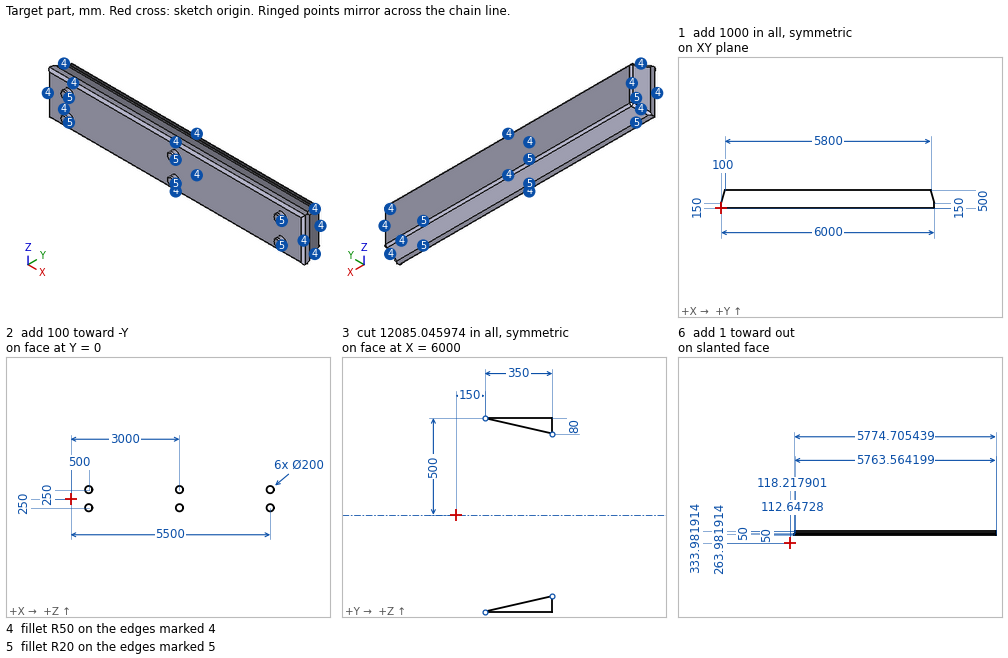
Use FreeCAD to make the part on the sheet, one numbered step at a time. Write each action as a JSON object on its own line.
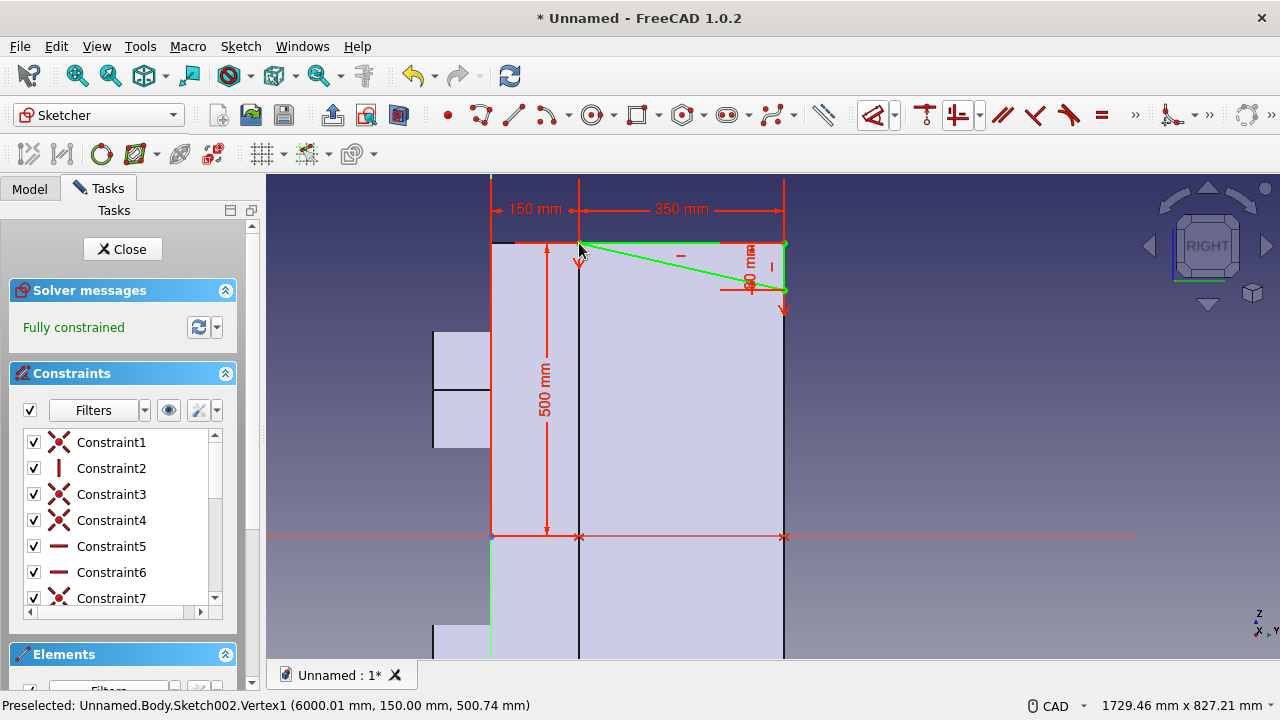
{"action": "left_click", "coordinate": [123, 249]}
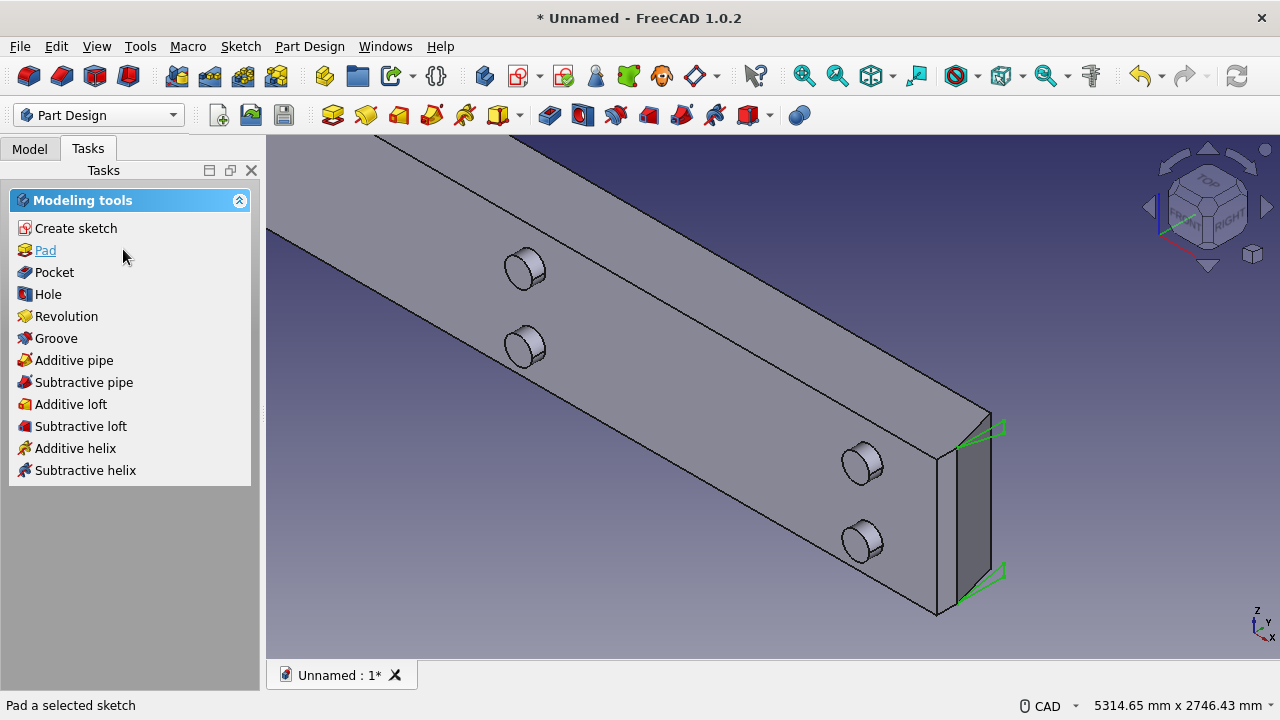
{"action": "left_click", "coordinate": [550, 116]}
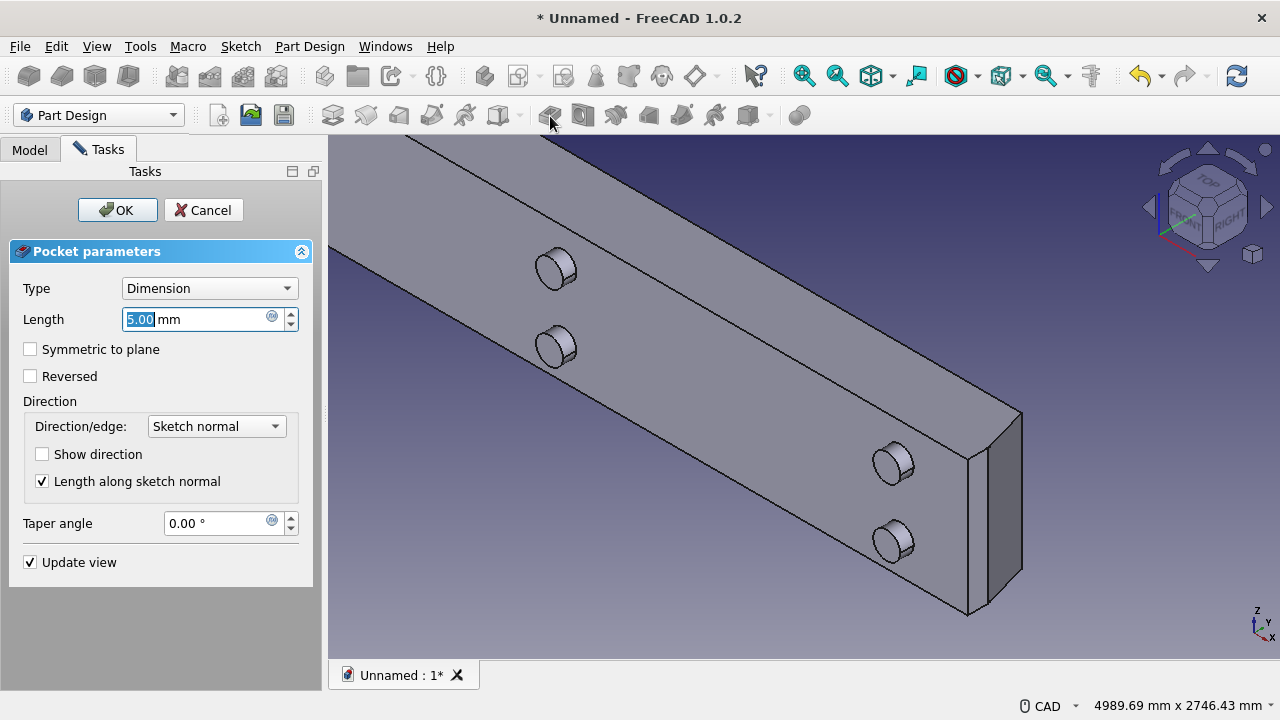
{"action": "type", "text": "12085.045974"}
{"action": "key", "text": "Tab"}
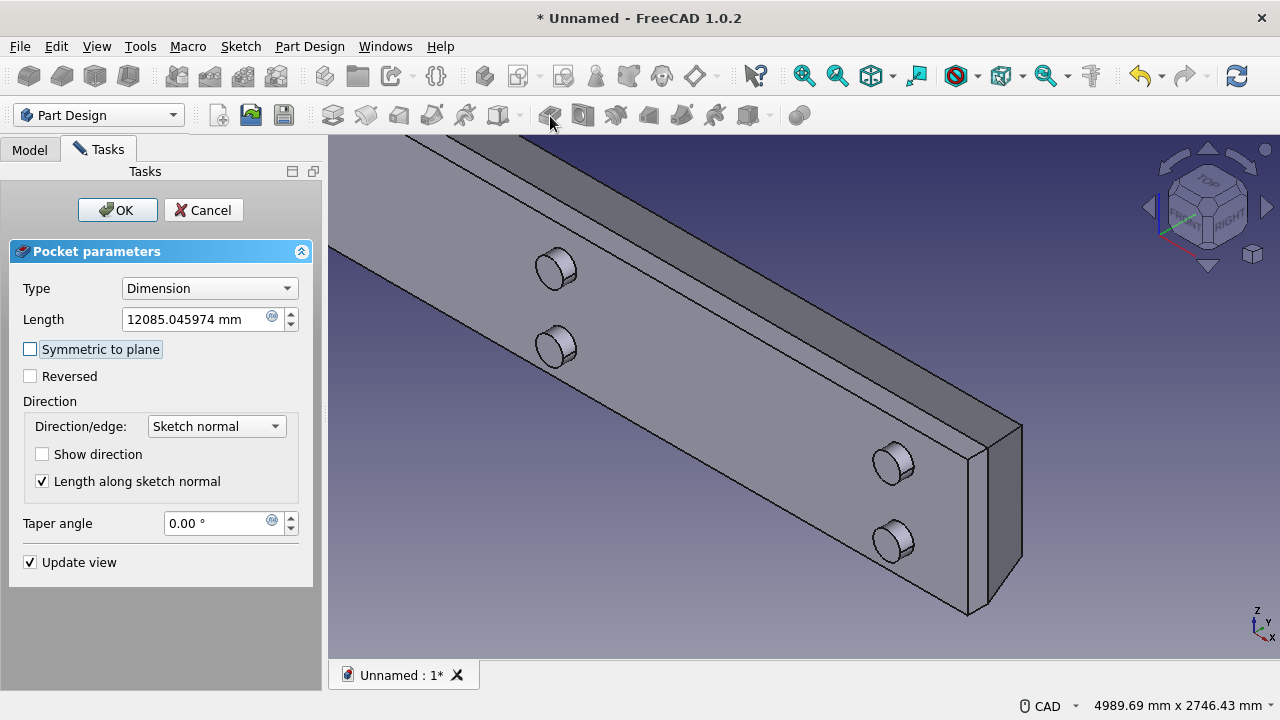
{"action": "left_click", "coordinate": [31, 349]}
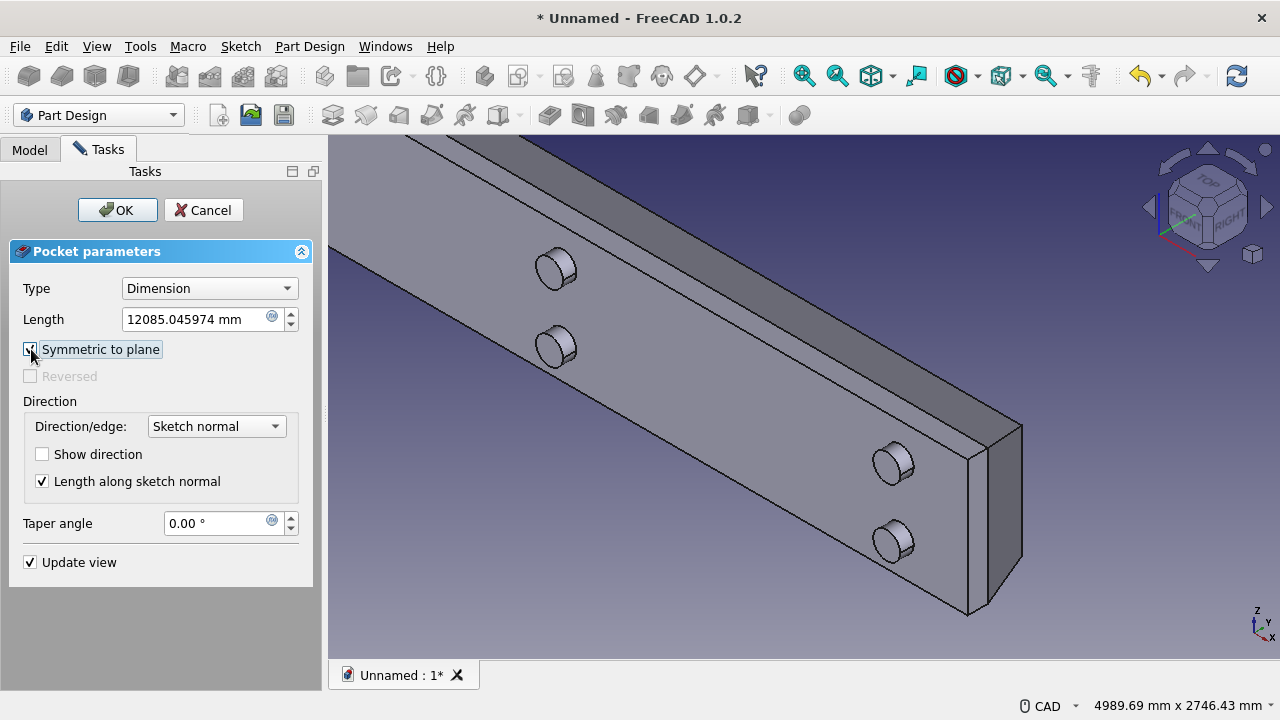
{"action": "left_click", "coordinate": [118, 210]}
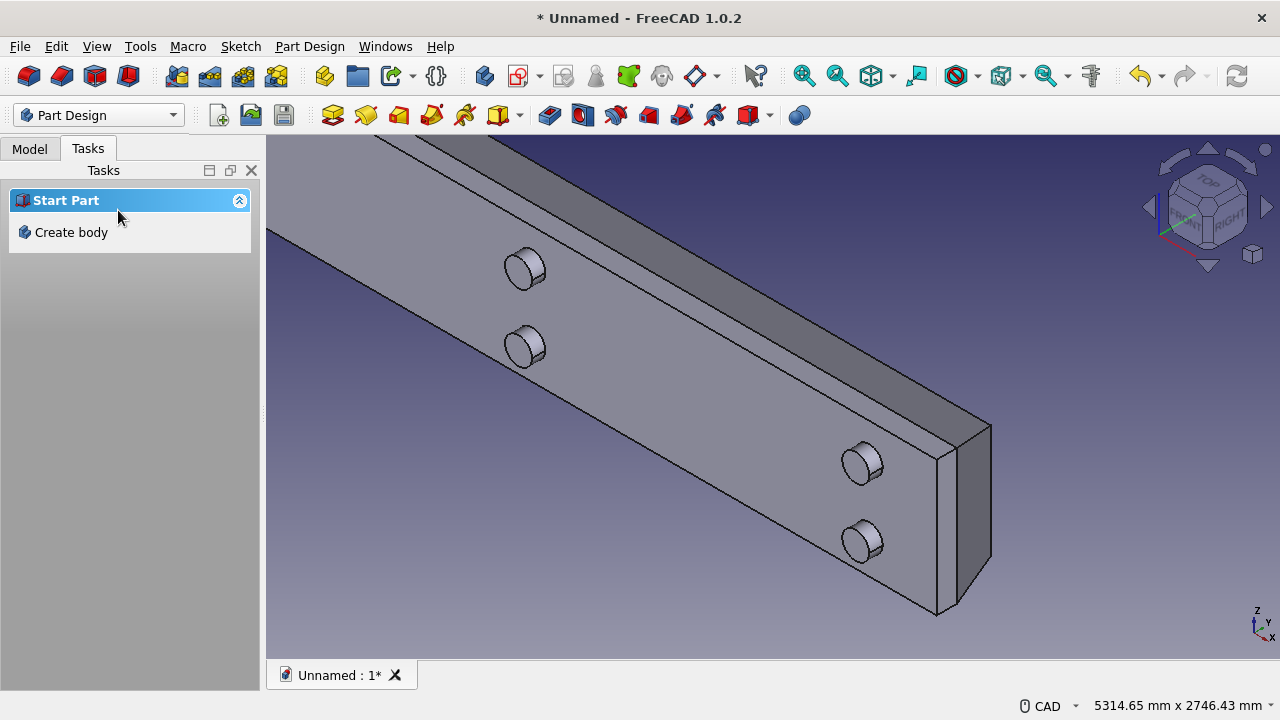
{"action": "left_click", "coordinate": [805, 76]}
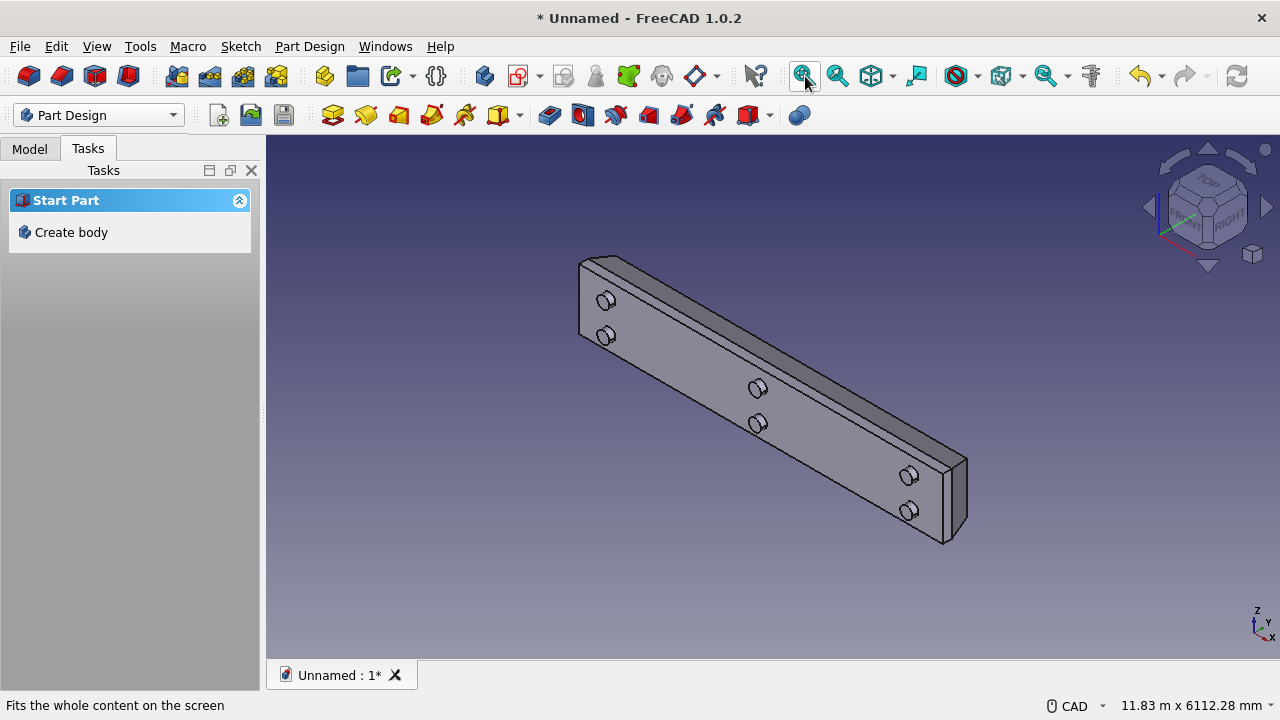
{"action": "left_click", "coordinate": [943, 508]}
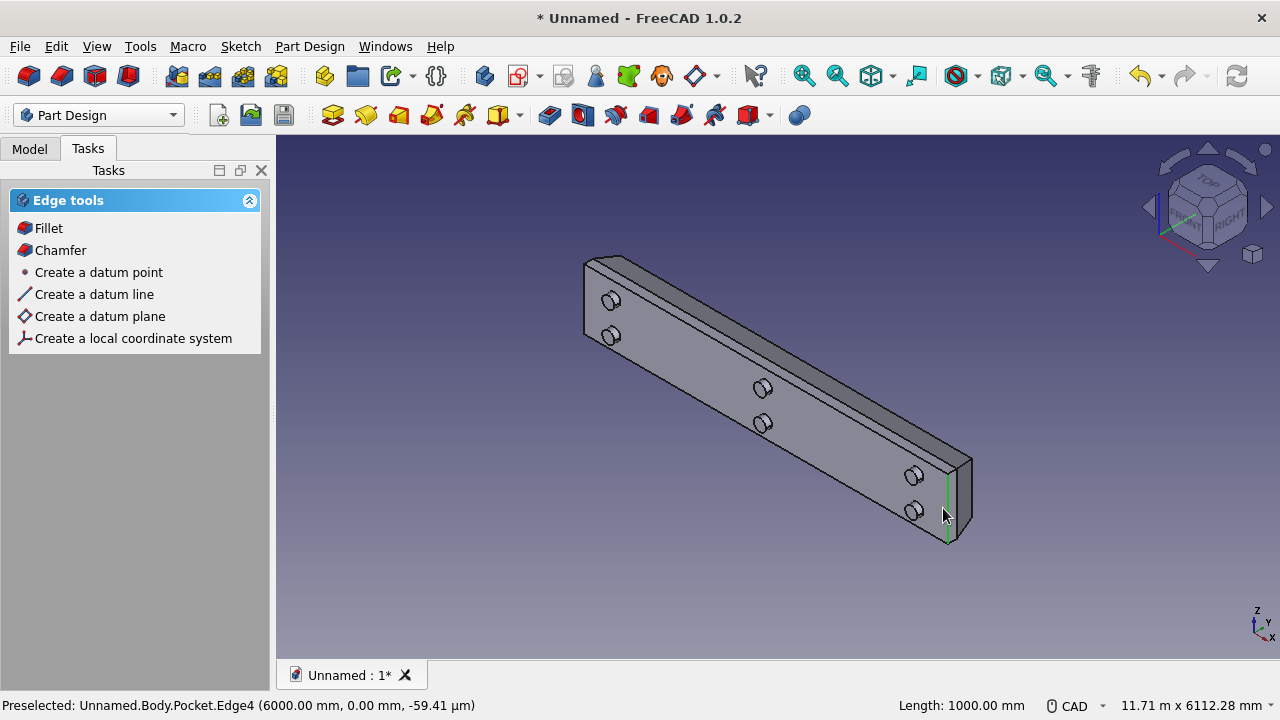
{"action": "left_click", "coordinate": [766, 368], "text": "ctrl"}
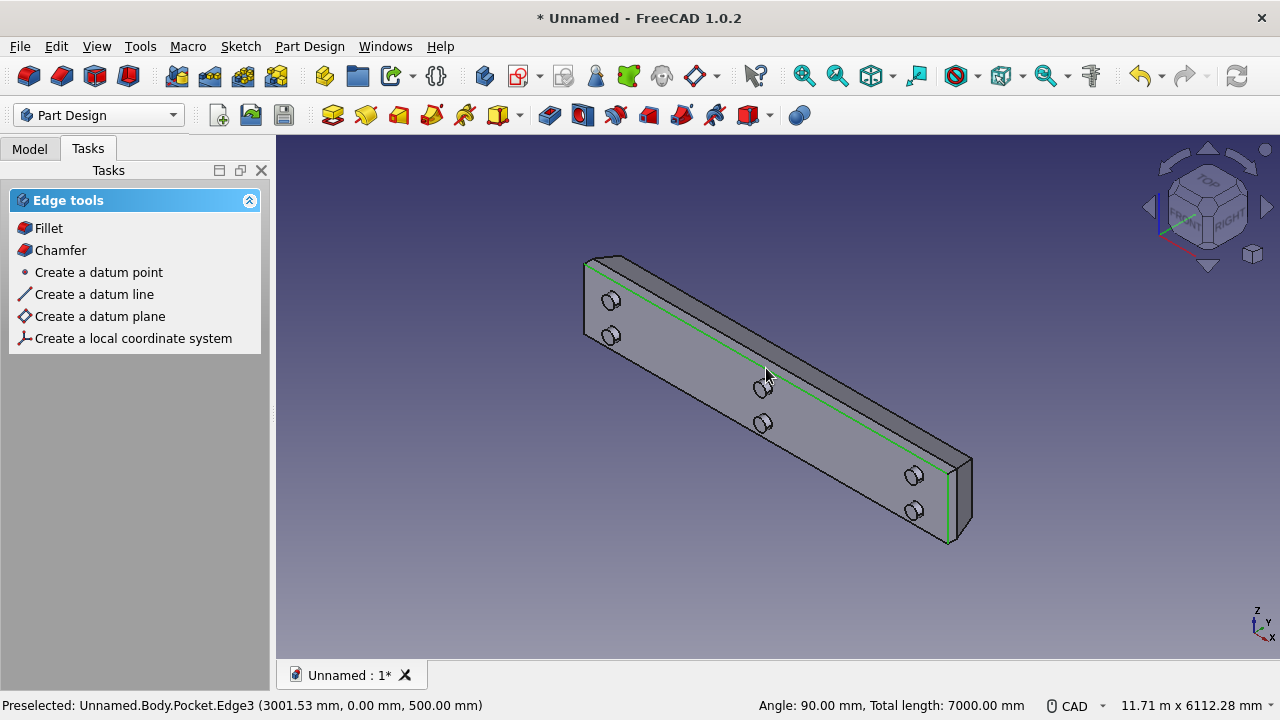
{"action": "left_click", "coordinate": [964, 463], "text": "ctrl"}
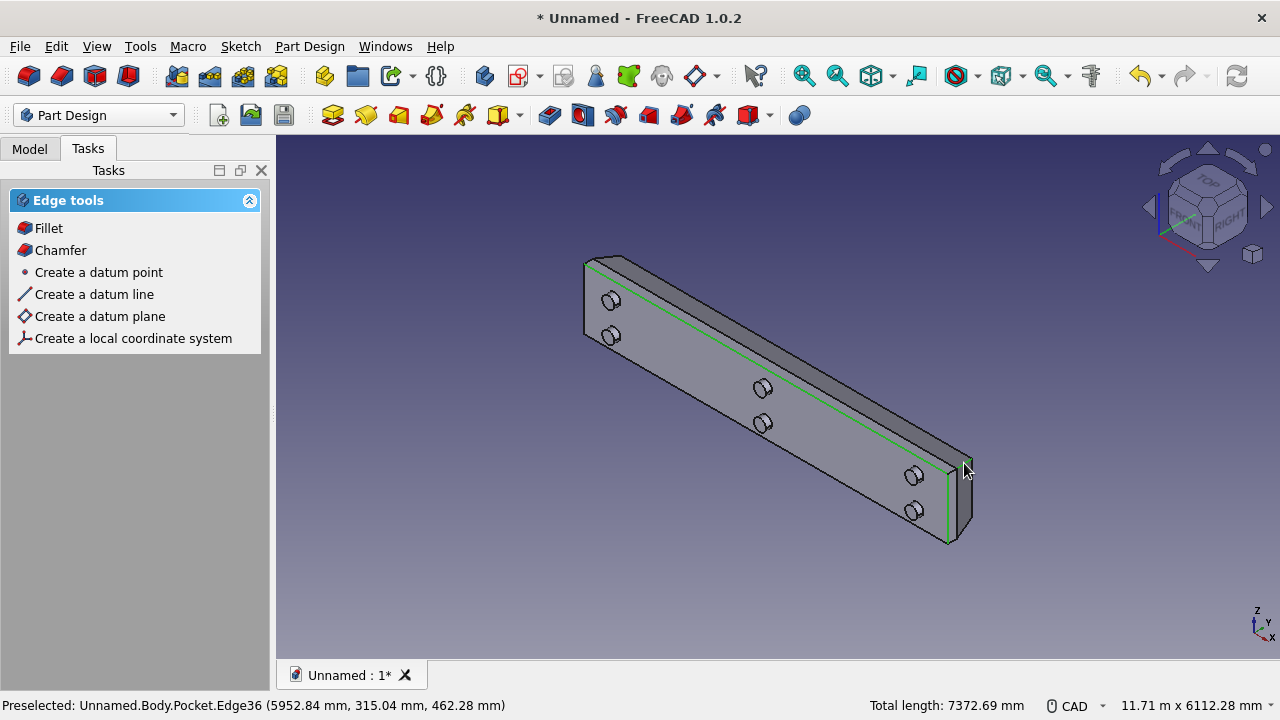
{"action": "key", "text": "2"}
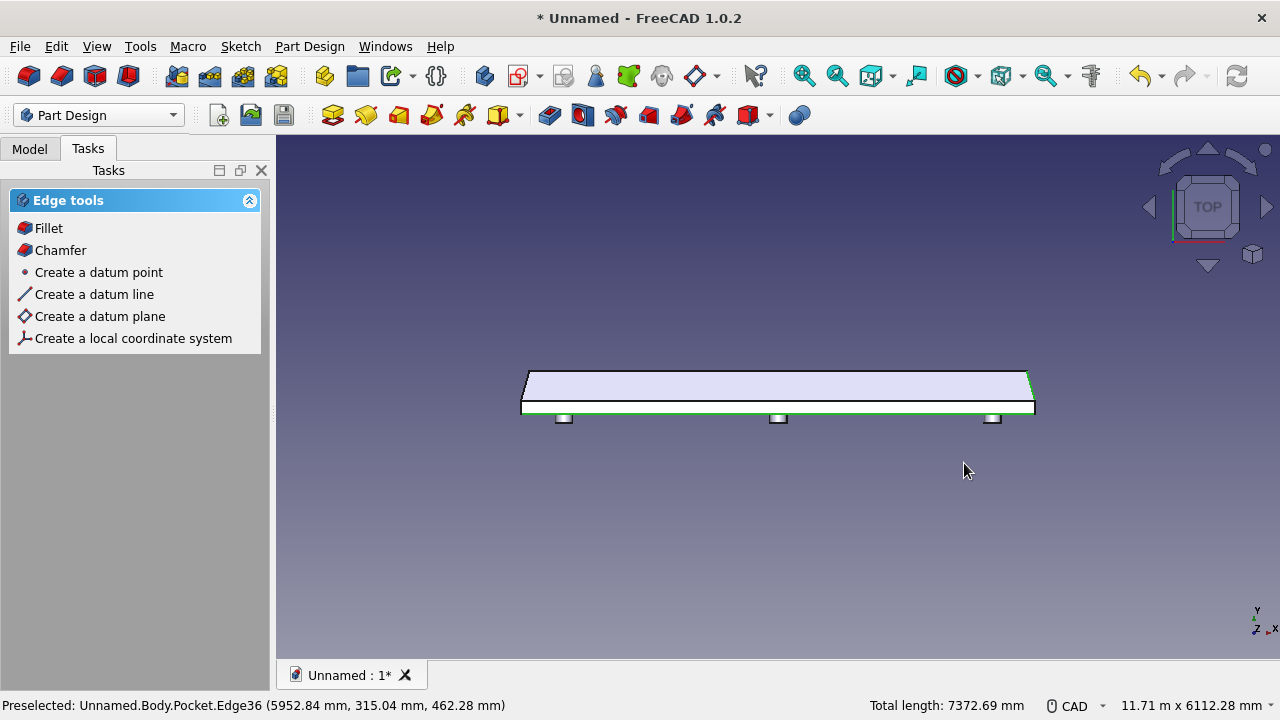
{"action": "key", "text": "0"}